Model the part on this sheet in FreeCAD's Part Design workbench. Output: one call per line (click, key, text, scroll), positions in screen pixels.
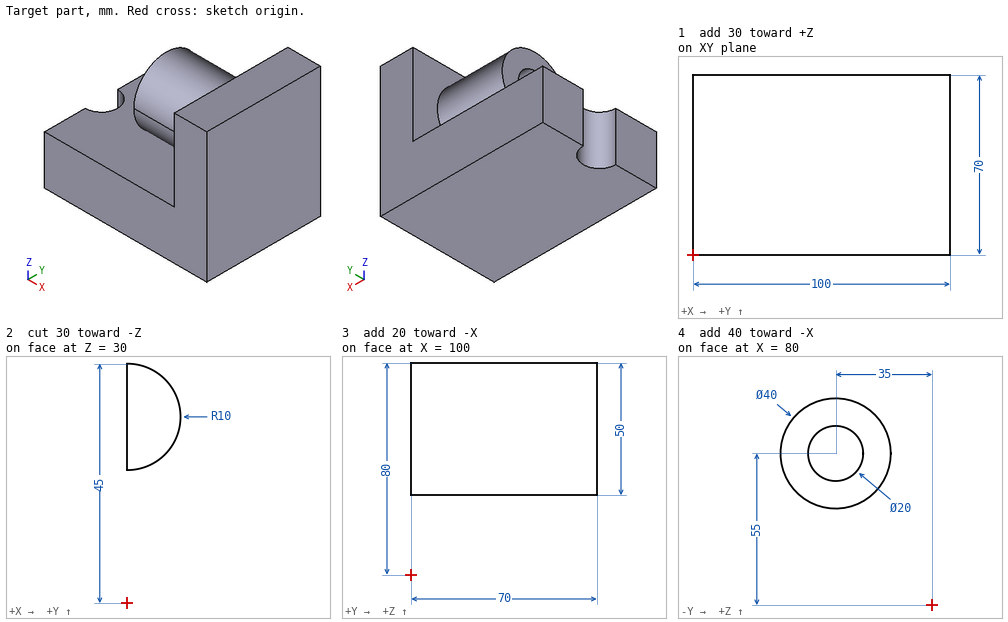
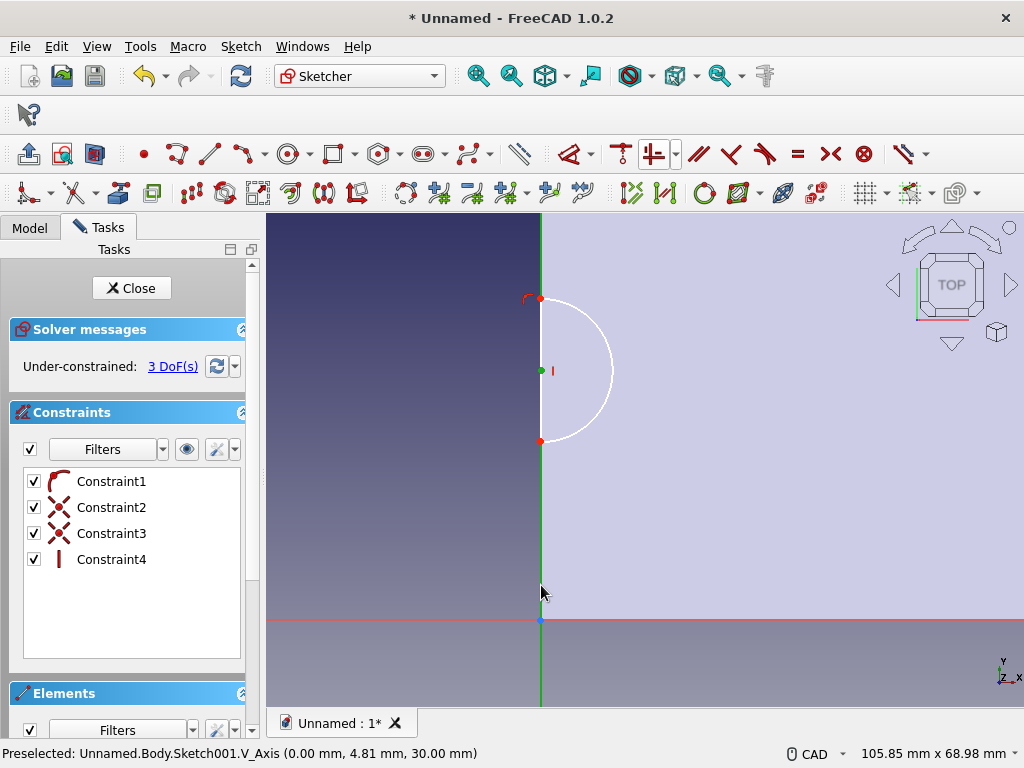
click(621, 154)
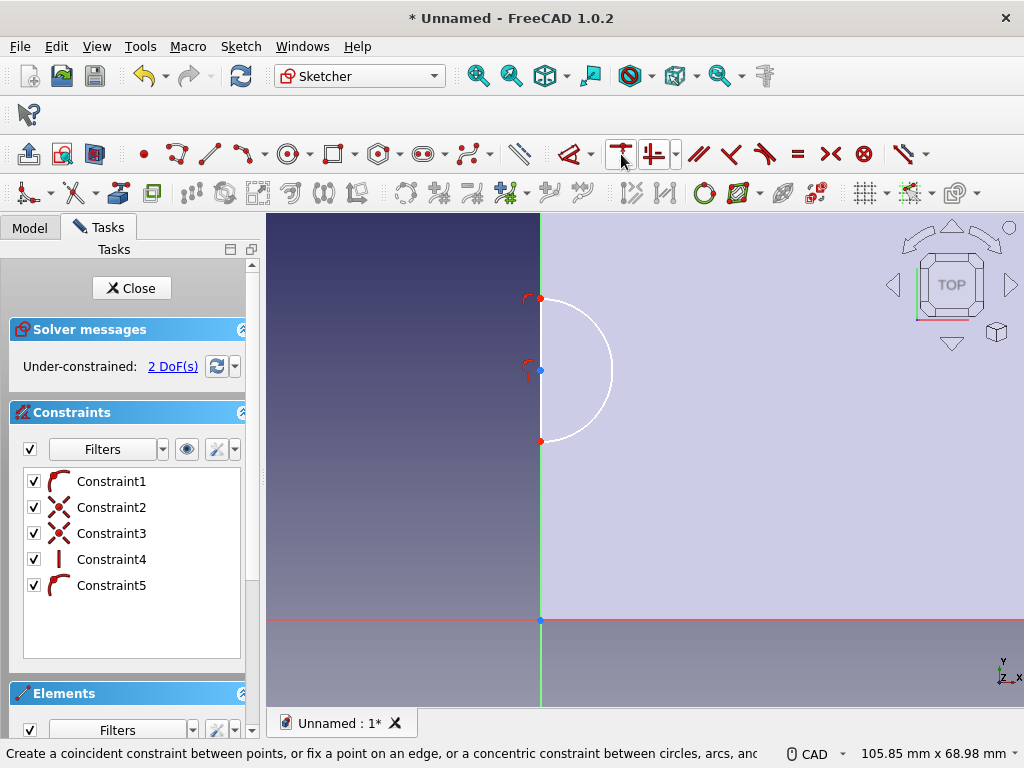
click(568, 154)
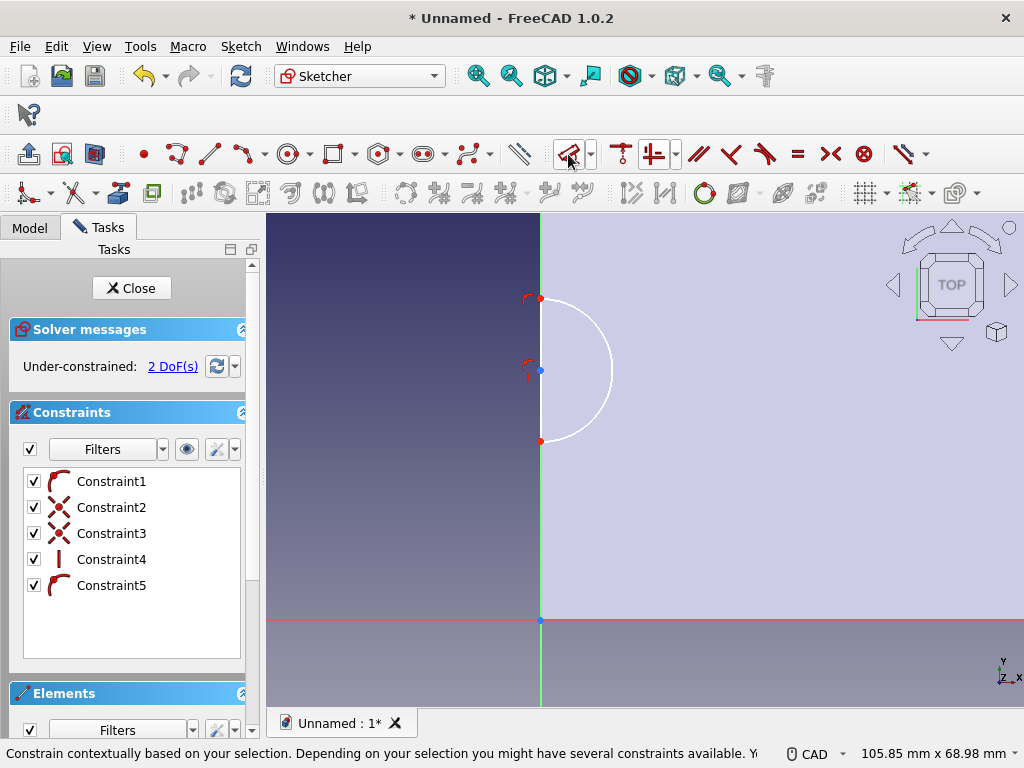
click(599, 413)
click(625, 432)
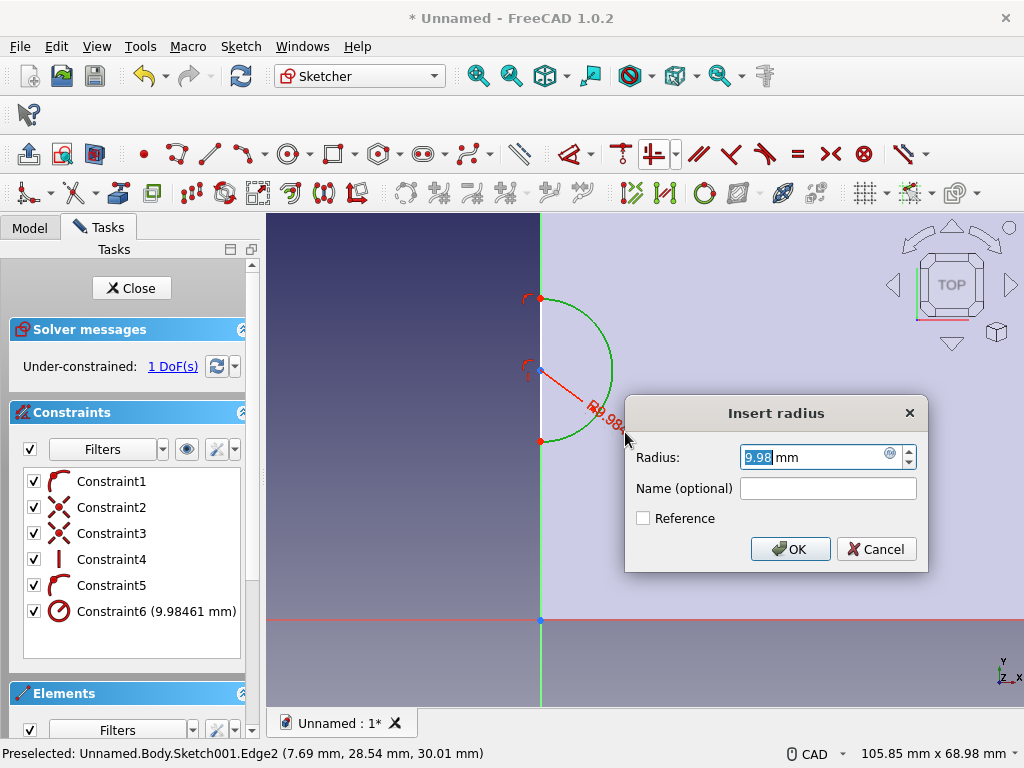
text(10)
key(Return)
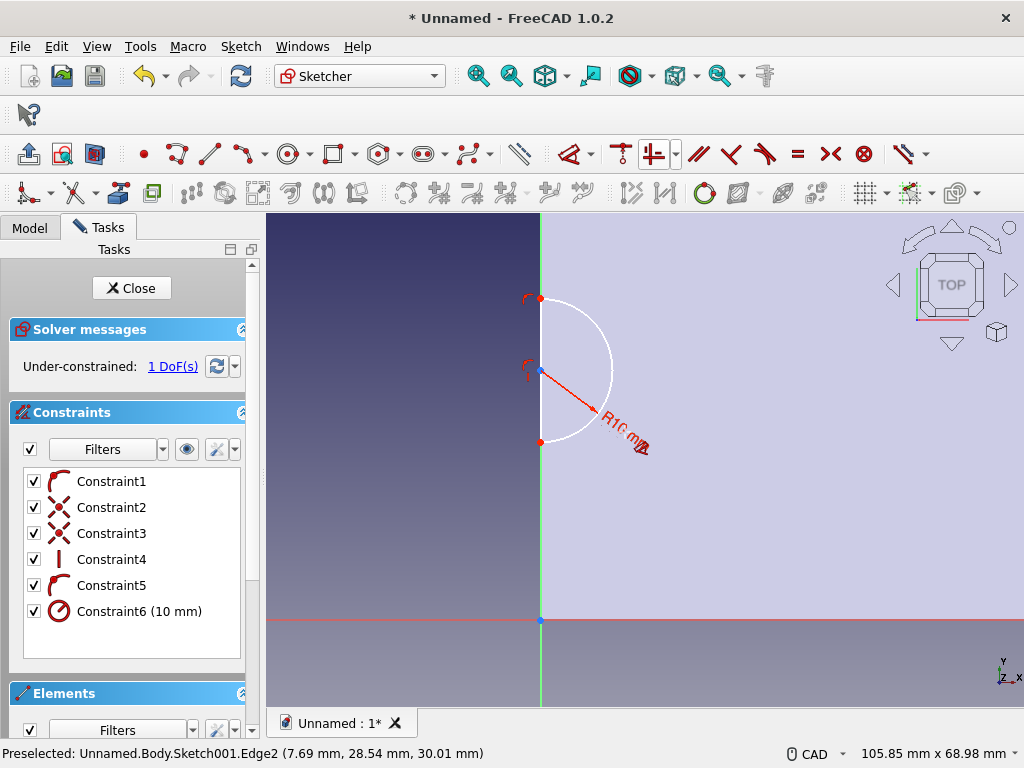
click(541, 299)
click(507, 460)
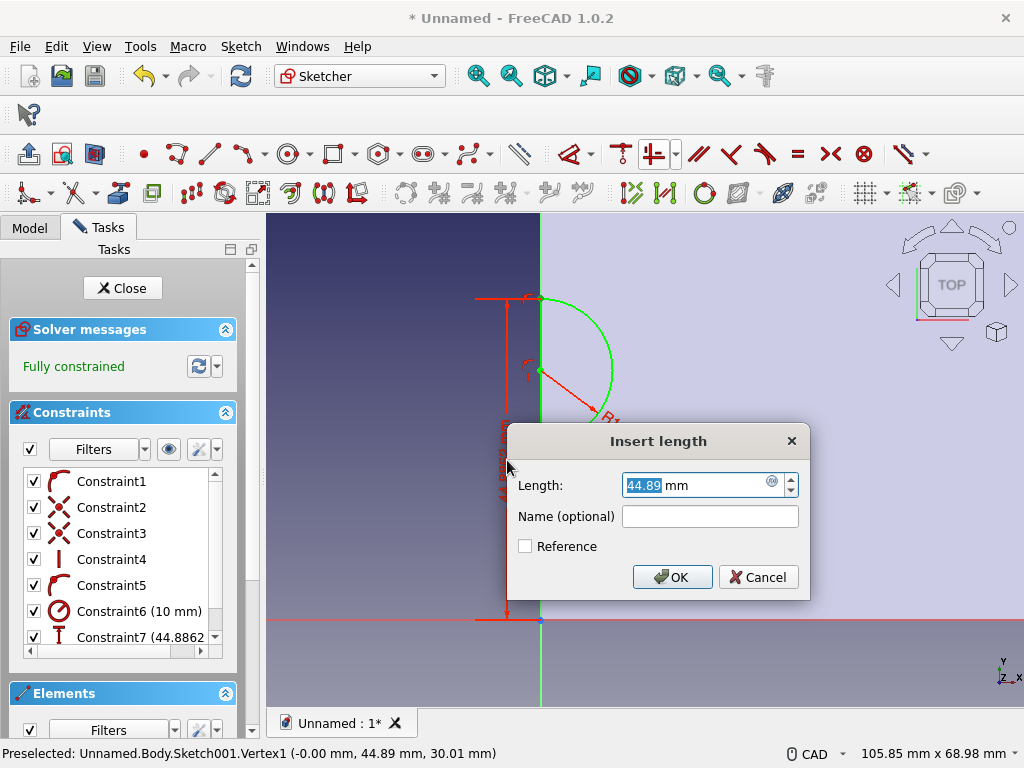
text(45)
key(Return)
key(Escape)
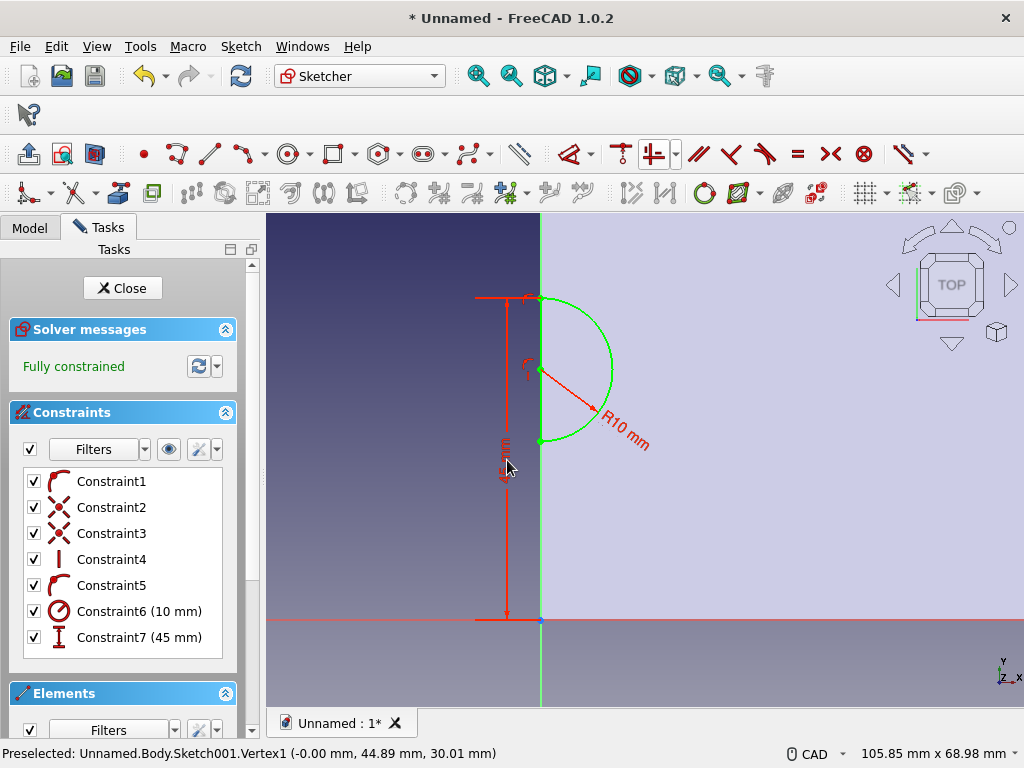
click(123, 288)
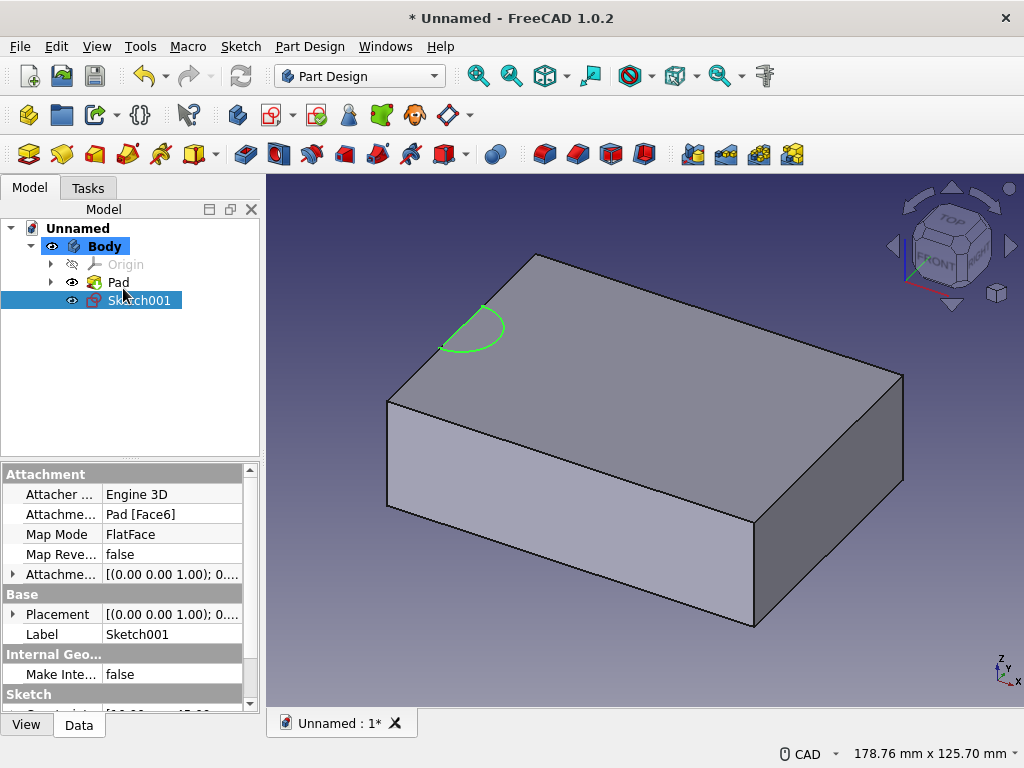
click(246, 154)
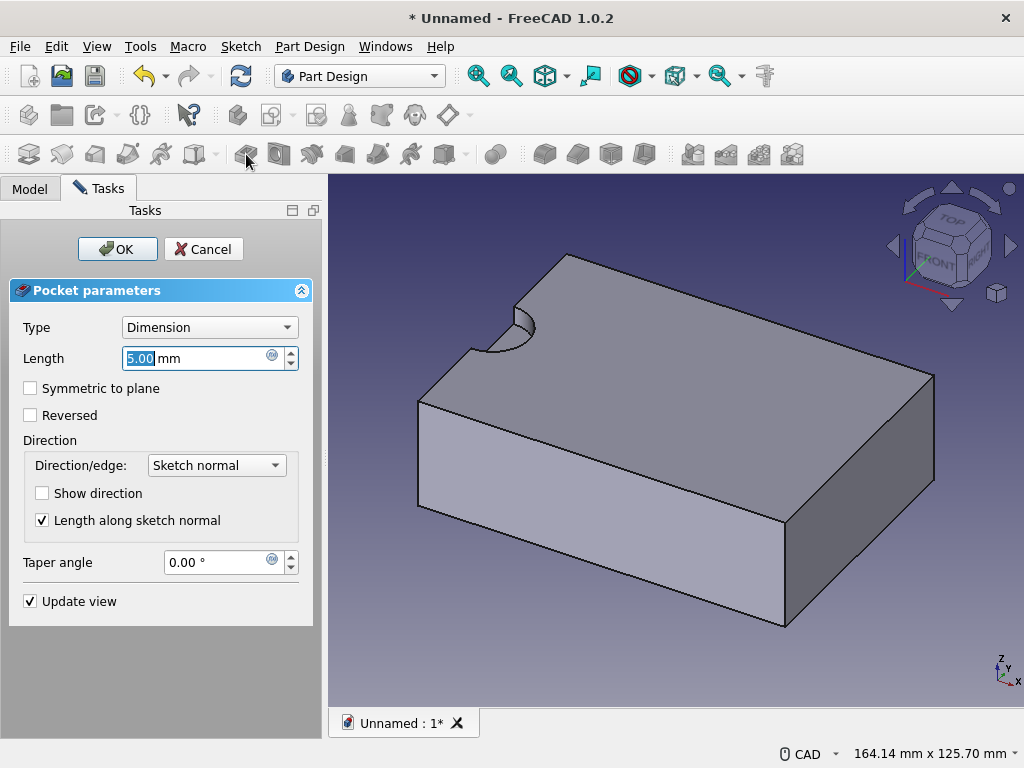
text(30)
key(Tab)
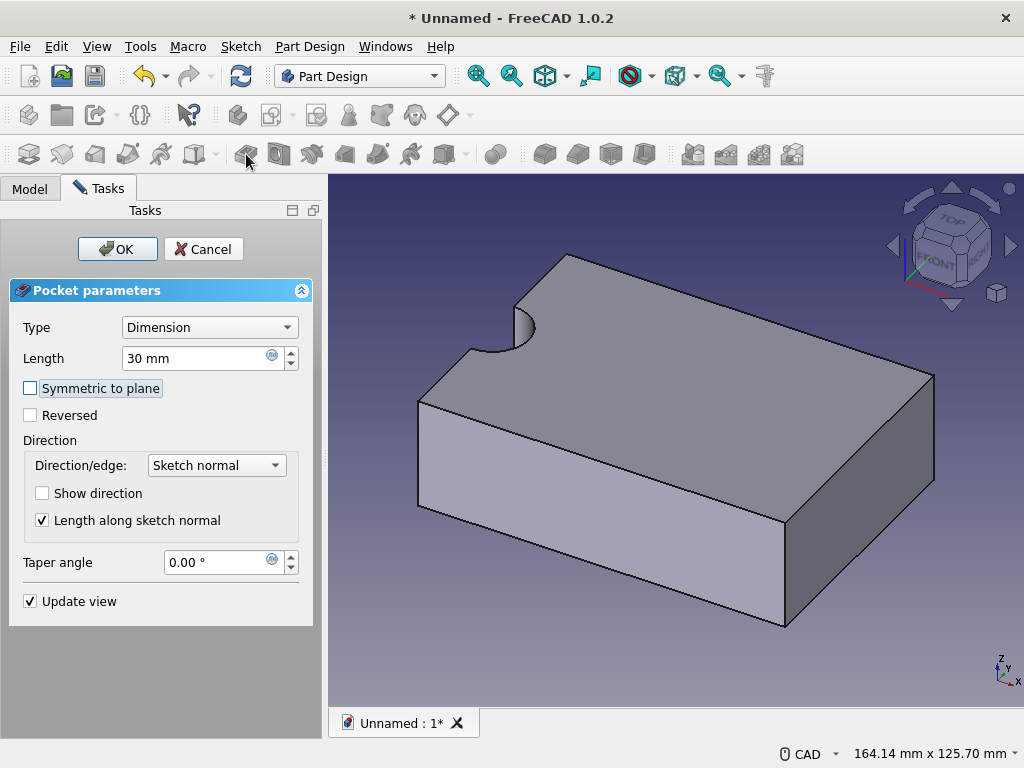
click(118, 249)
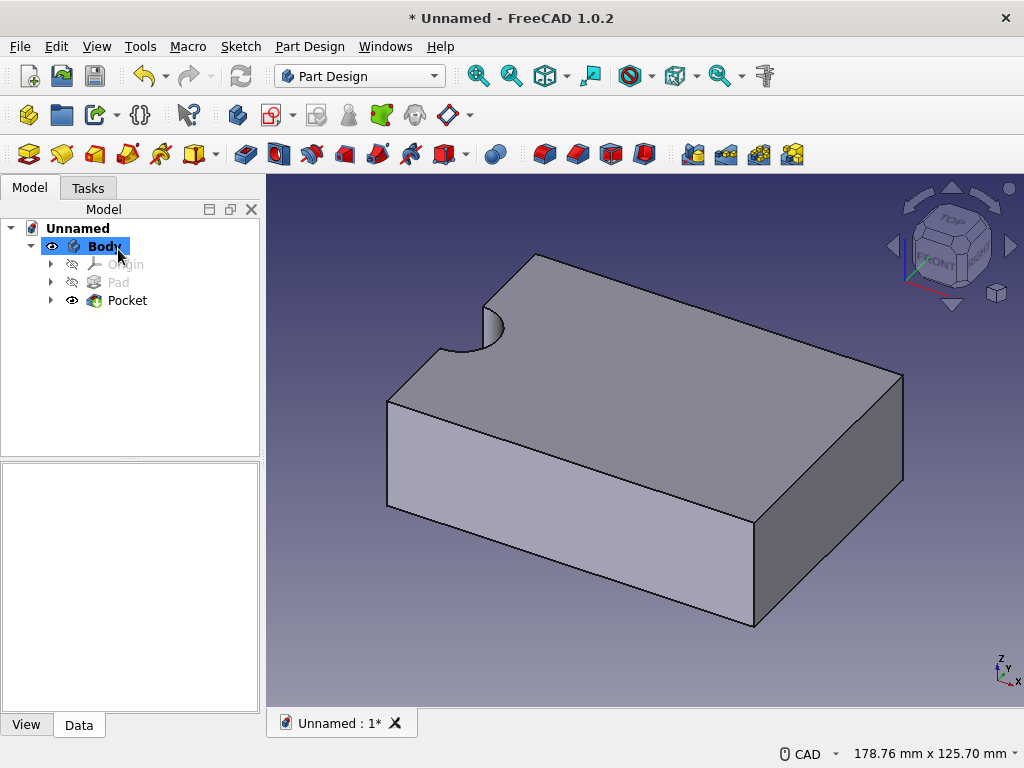
click(871, 458)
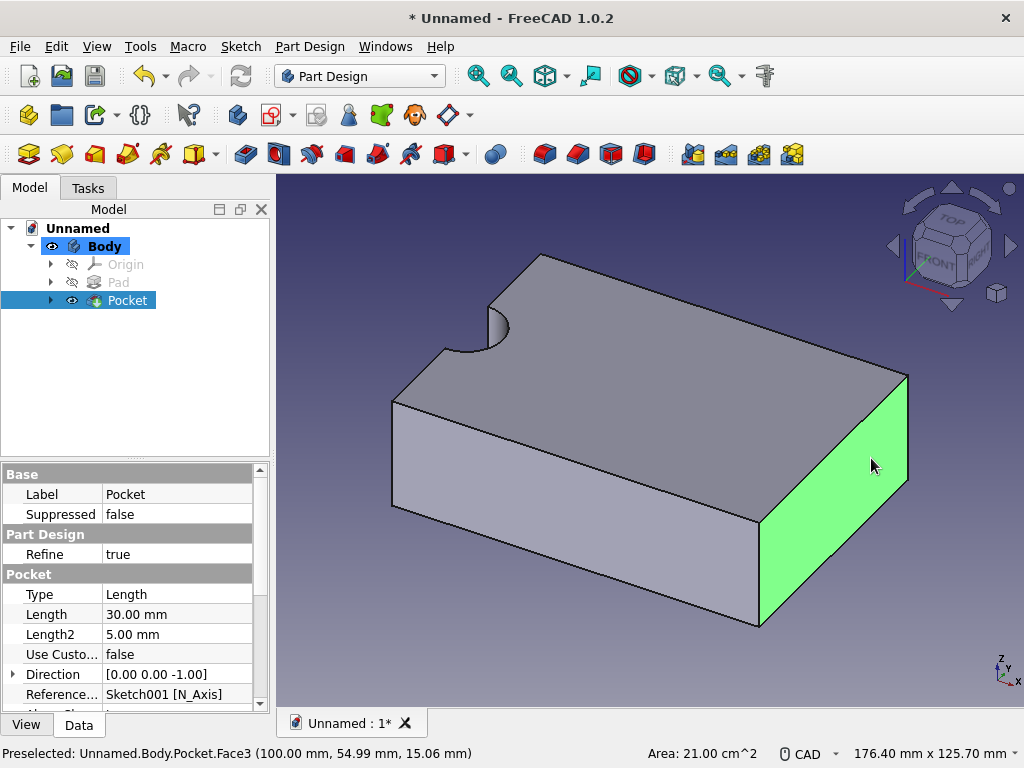
click(270, 116)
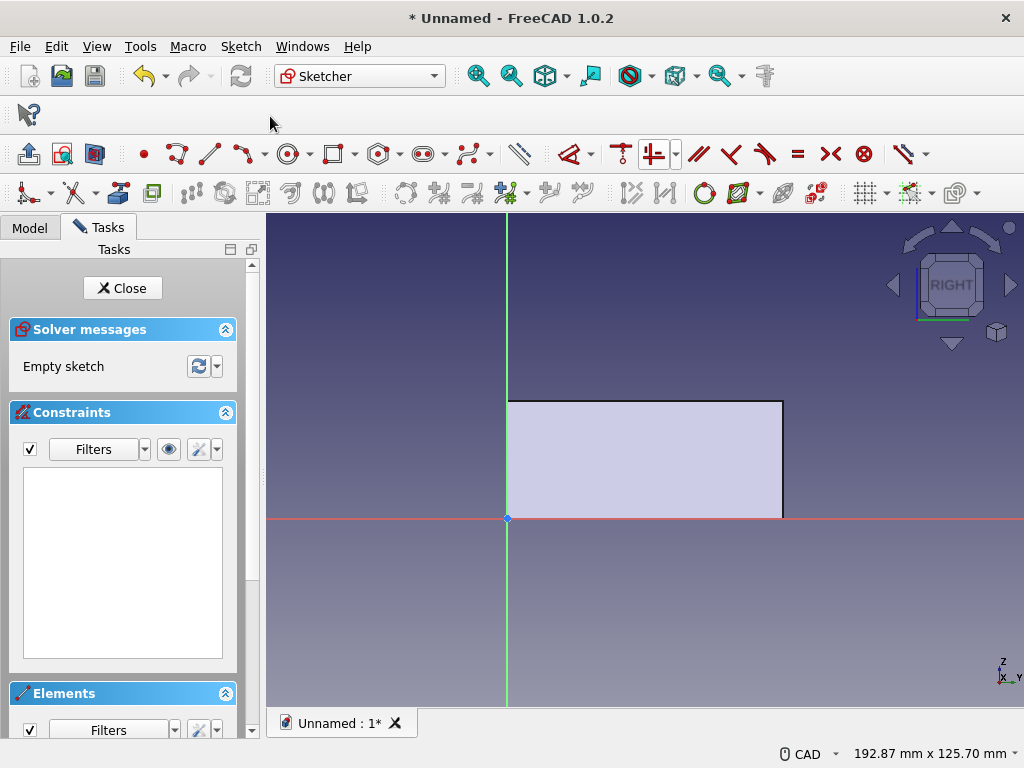
scroll(294, 679, down, 1)